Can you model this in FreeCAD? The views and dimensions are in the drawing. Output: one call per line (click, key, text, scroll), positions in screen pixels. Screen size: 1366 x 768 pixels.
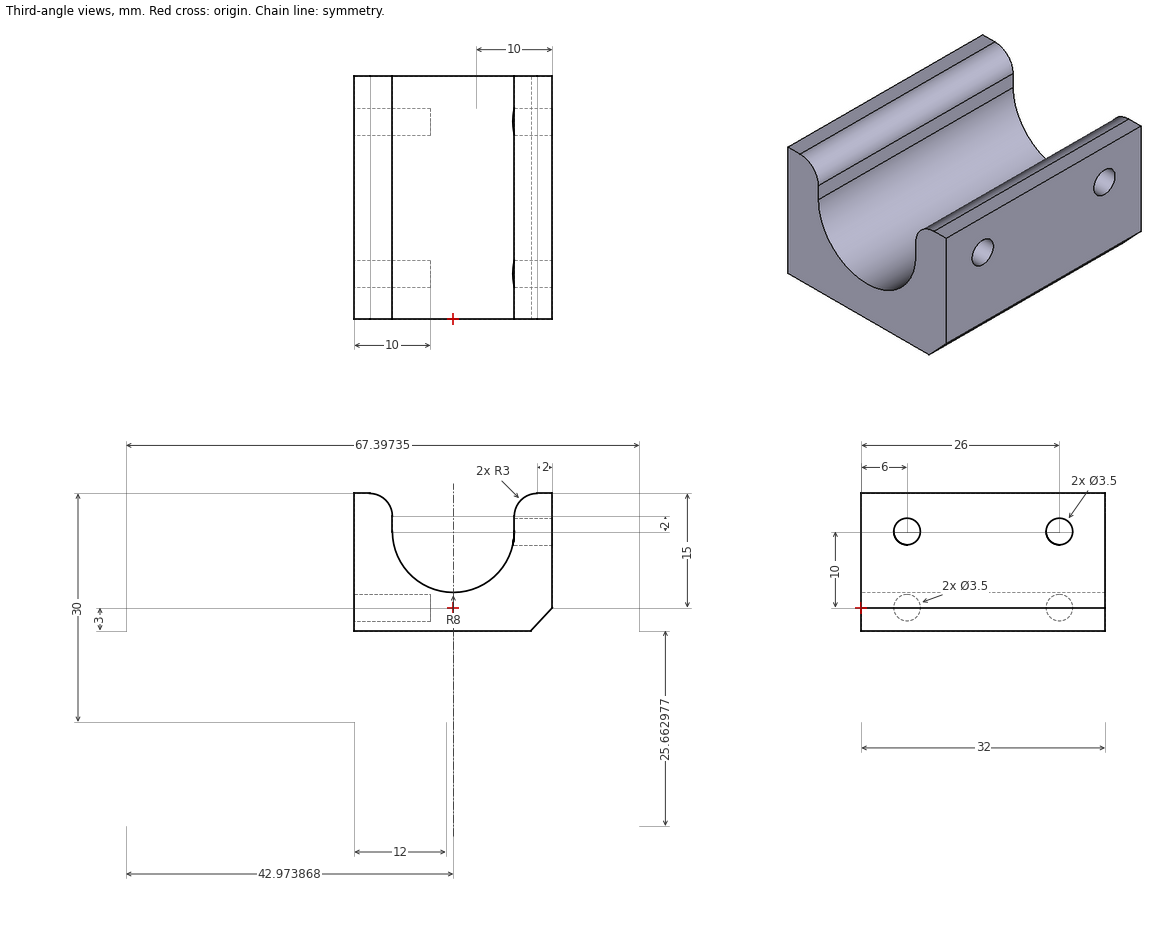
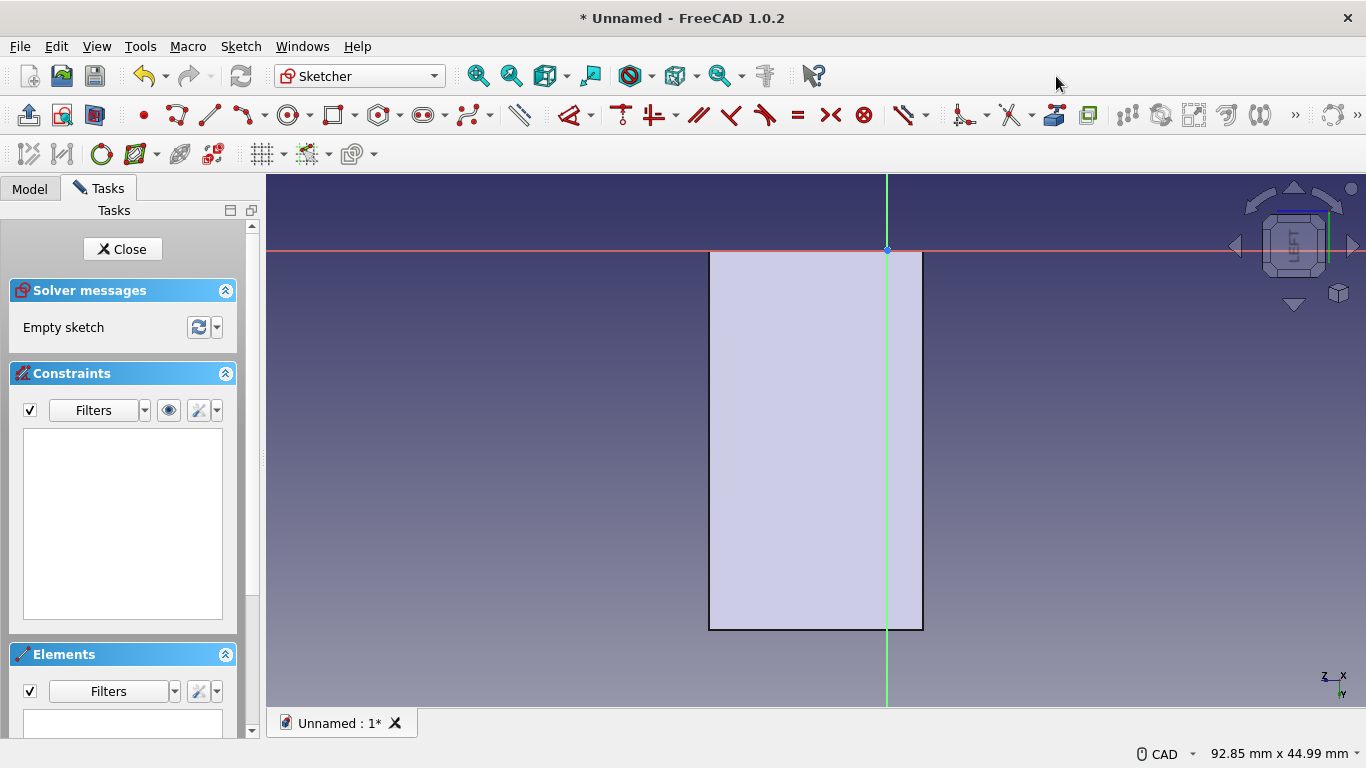
click(288, 116)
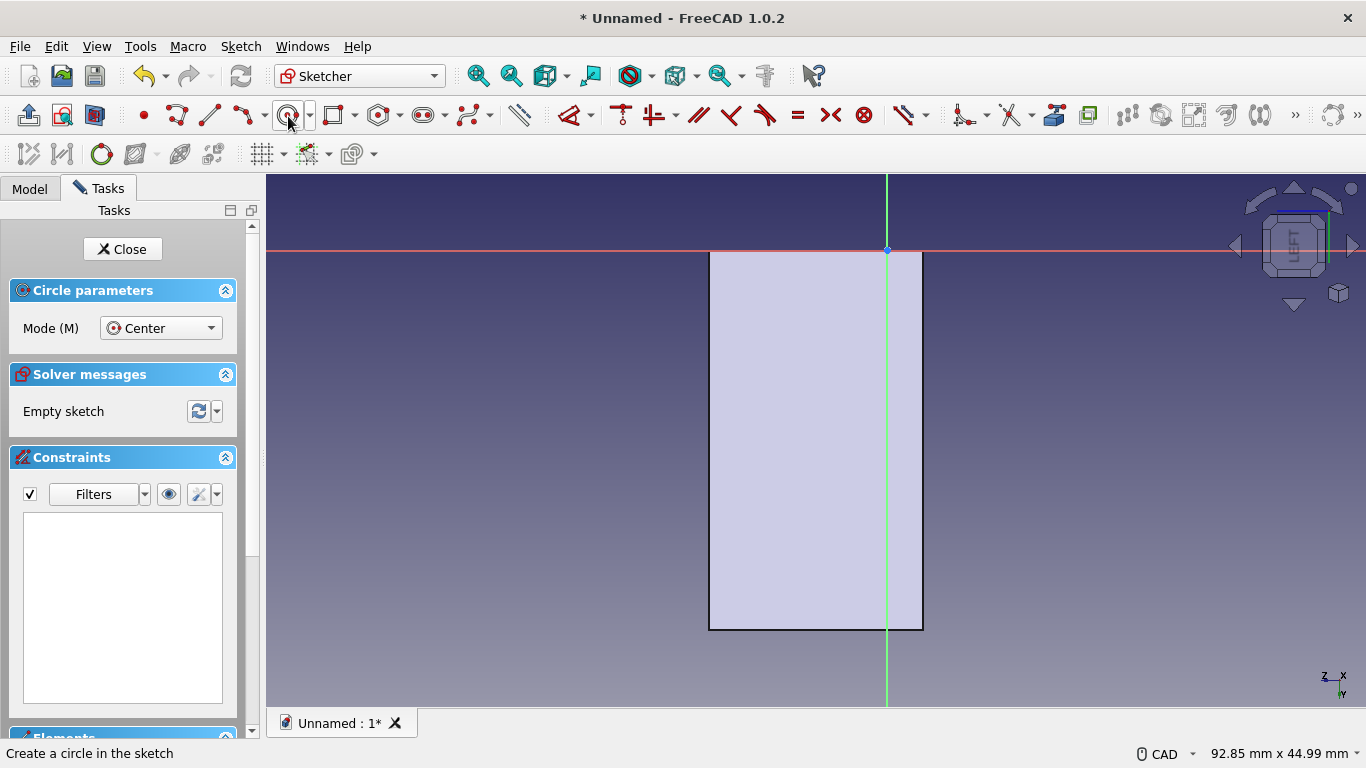
click(887, 322)
move(902, 307)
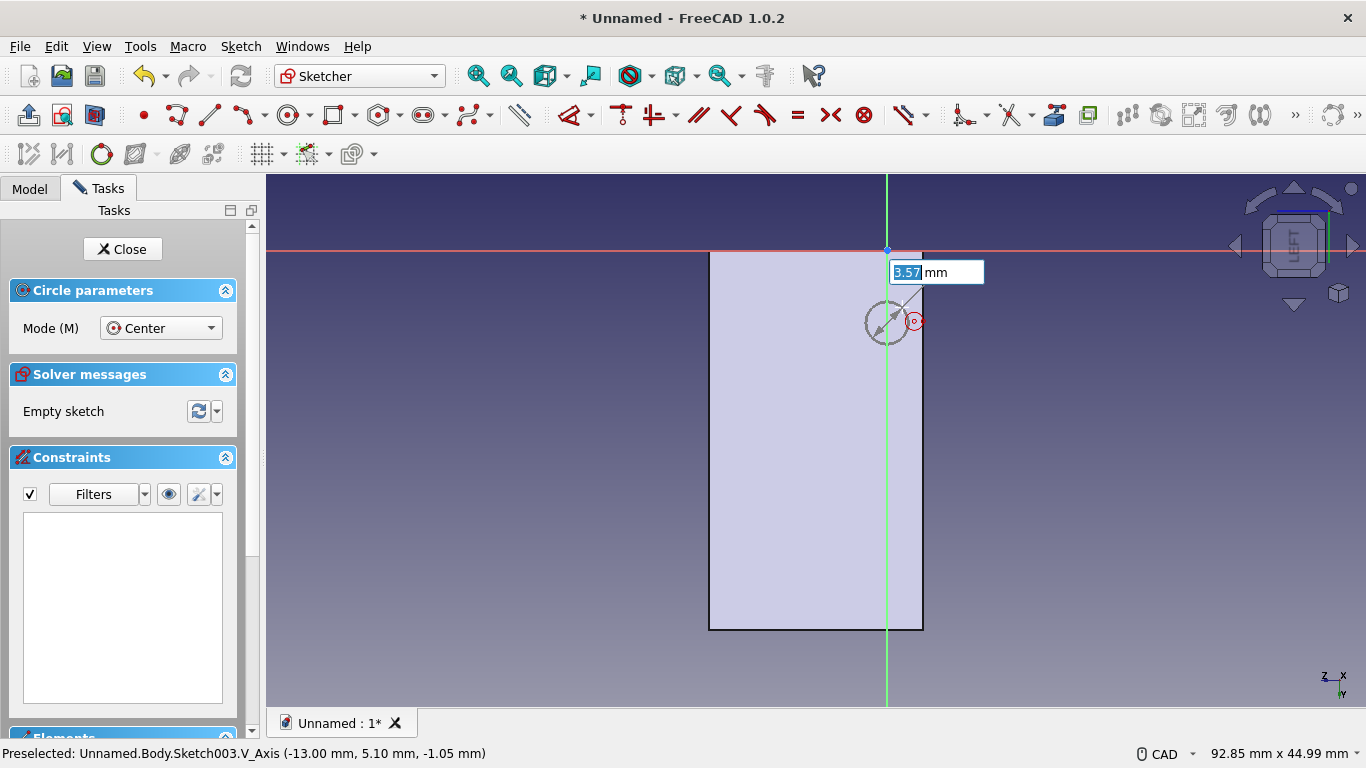
text(3.5)
key(Return)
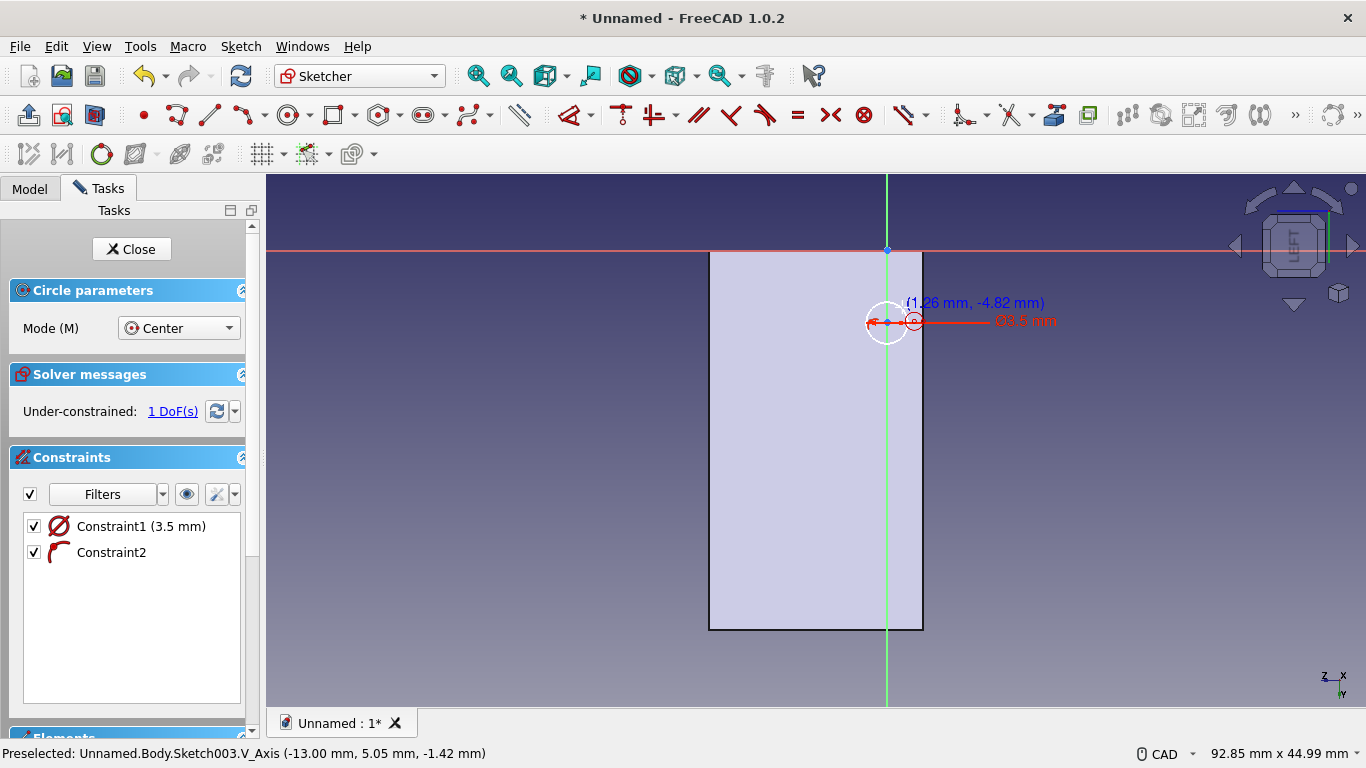
click(887, 559)
move(902, 544)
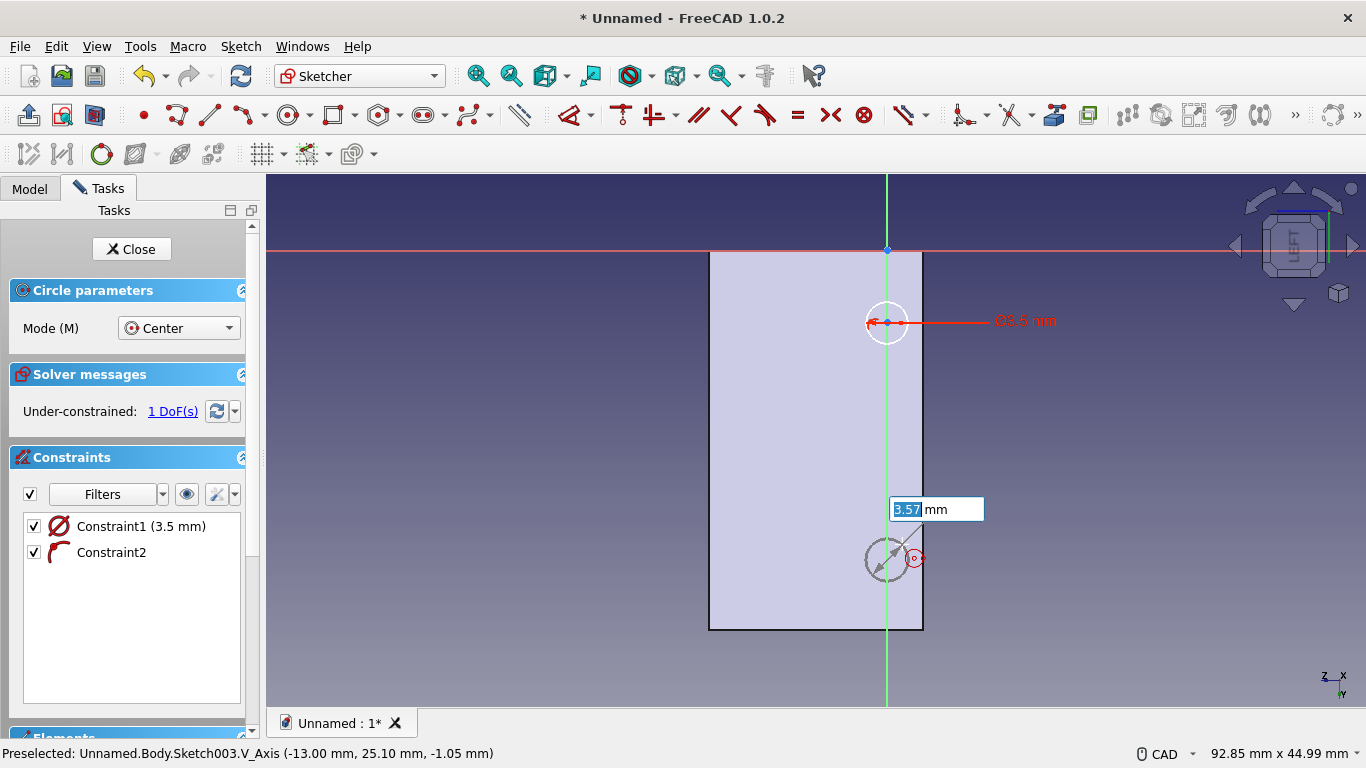
text(3.5)
key(Return)
key(Escape)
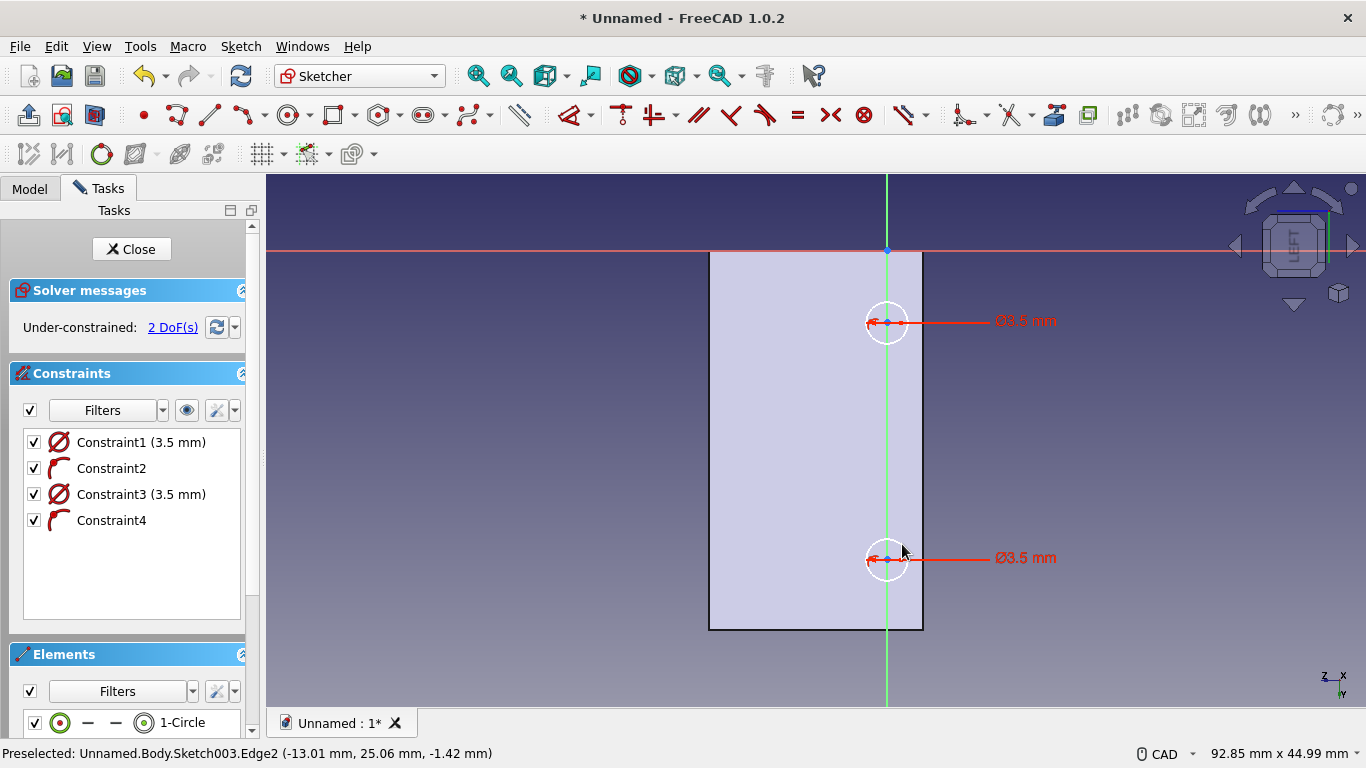
click(568, 116)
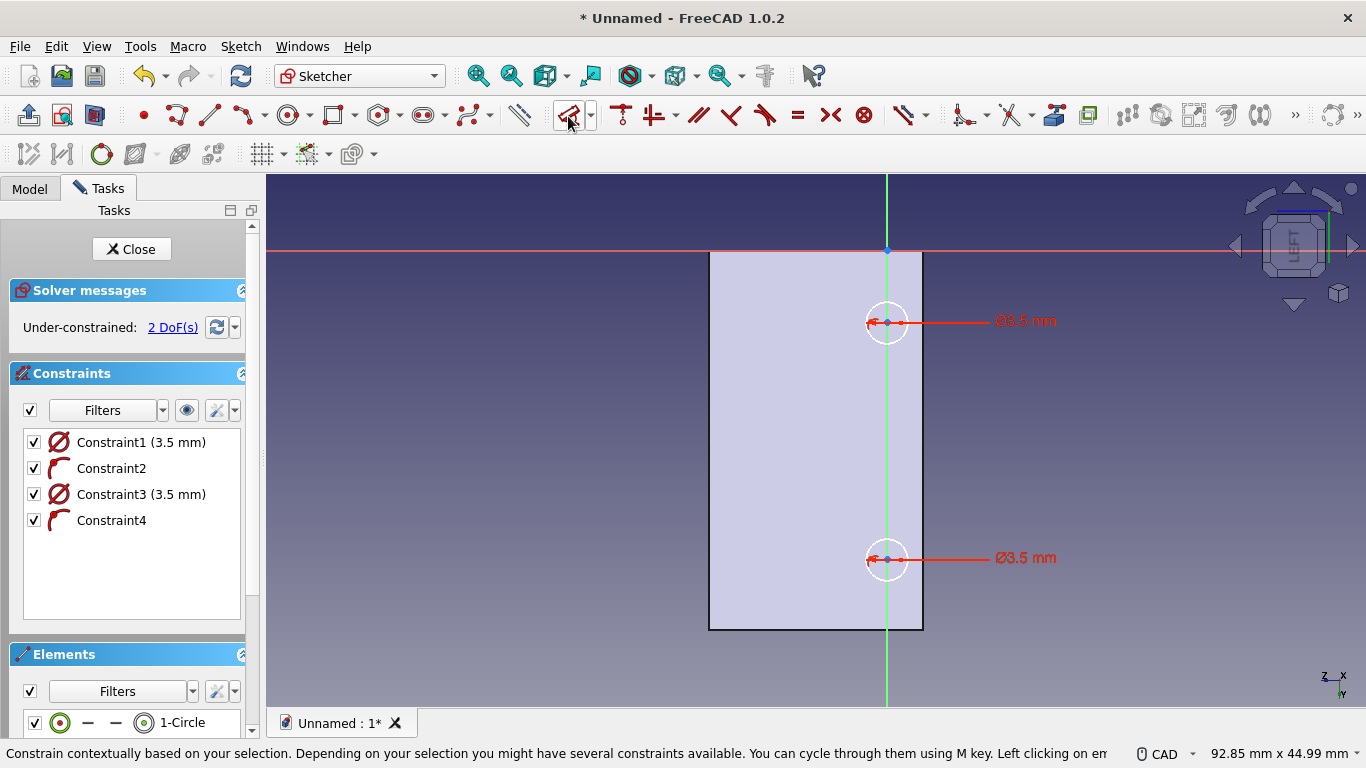
click(887, 323)
click(921, 287)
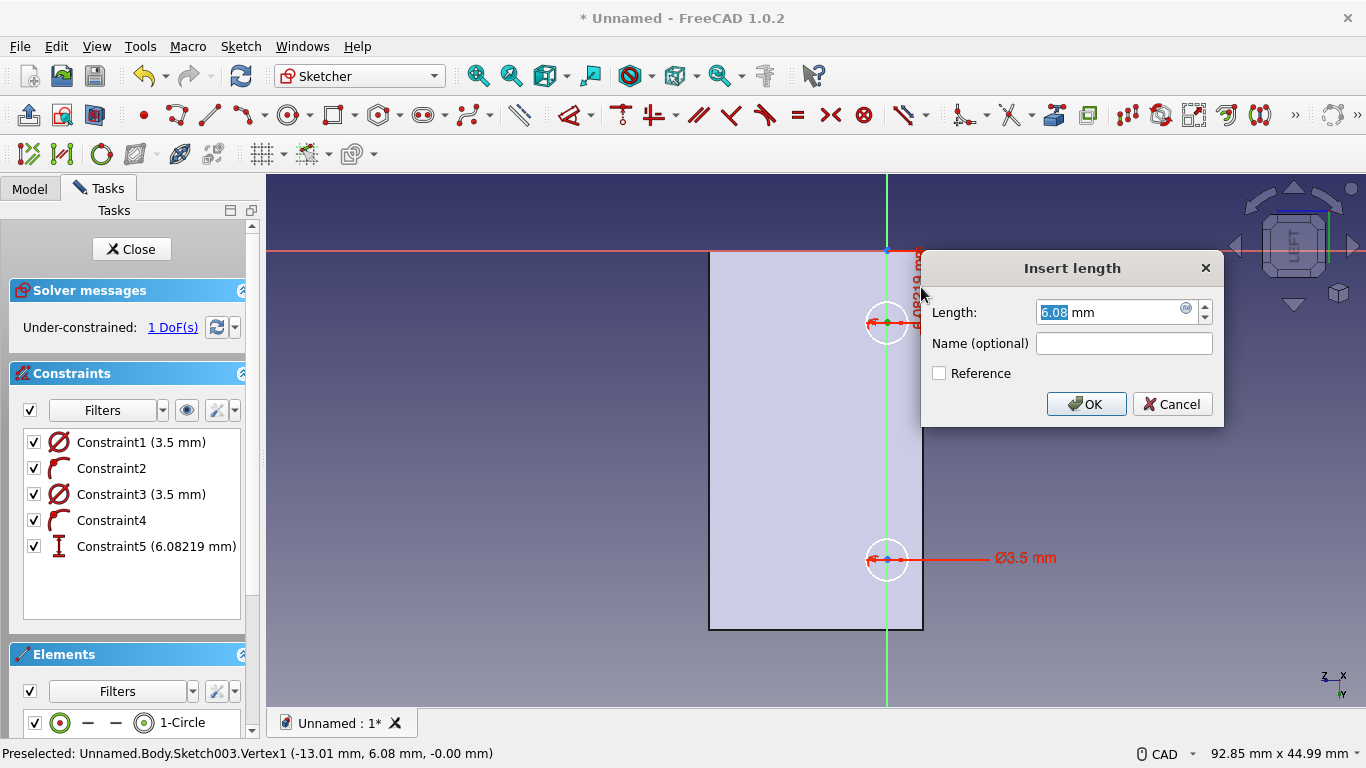
text(6)
key(Return)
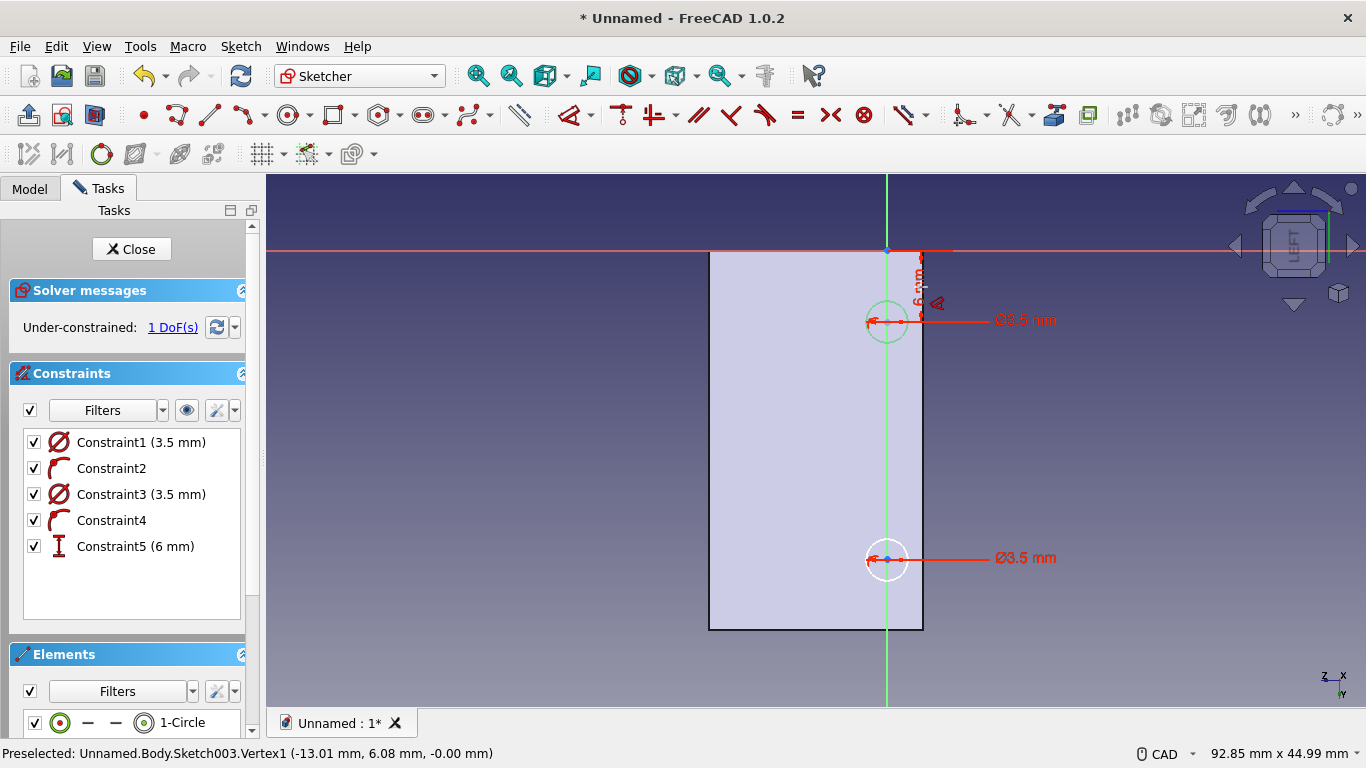
click(887, 560)
click(921, 405)